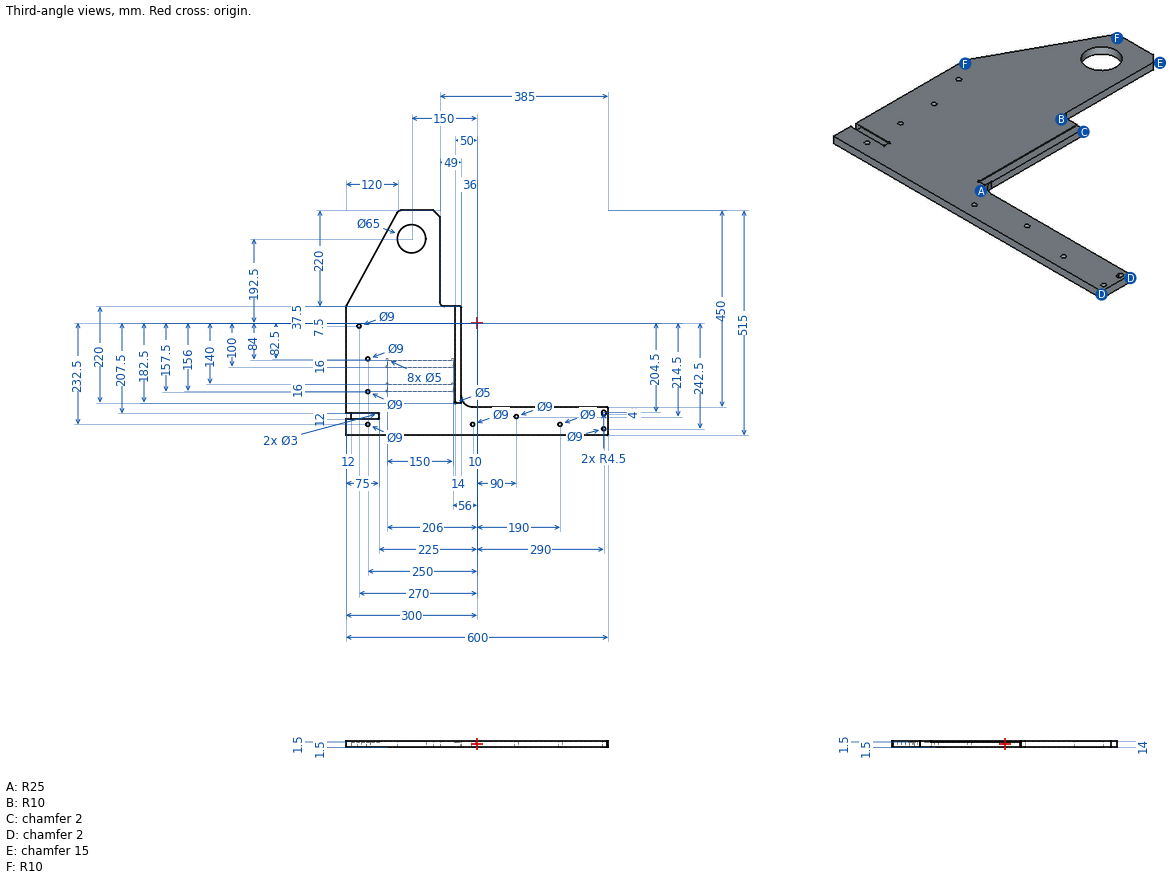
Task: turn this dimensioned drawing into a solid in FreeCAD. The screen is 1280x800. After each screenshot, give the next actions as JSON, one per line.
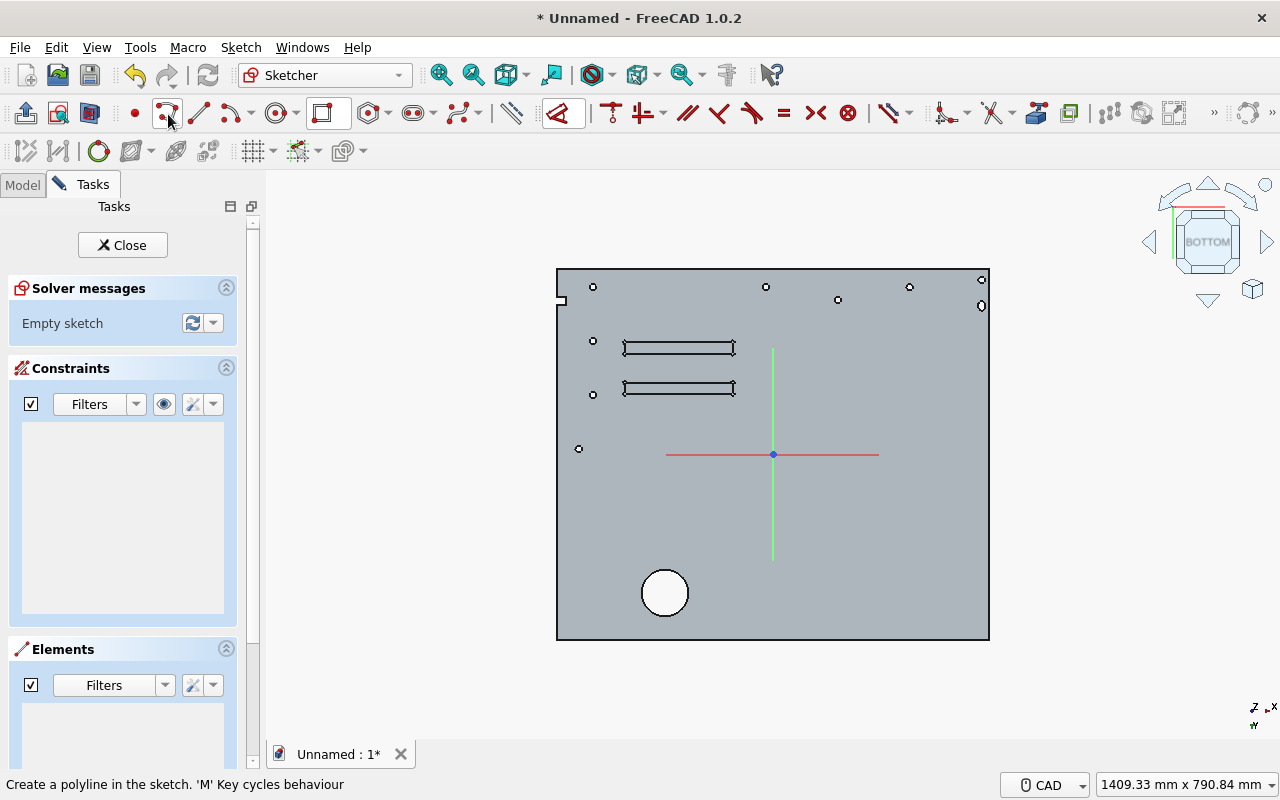
{"action": "left_click", "coordinate": [747, 481]}
{"action": "left_click", "coordinate": [712, 481]}
{"action": "left_click", "coordinate": [712, 640]}
{"action": "left_click", "coordinate": [989, 640]}
{"action": "left_click", "coordinate": [989, 316]}
{"action": "left_click", "coordinate": [747, 316]}
{"action": "left_click", "coordinate": [747, 482]}
{"action": "key", "text": "Escape"}
{"action": "key", "text": "Escape"}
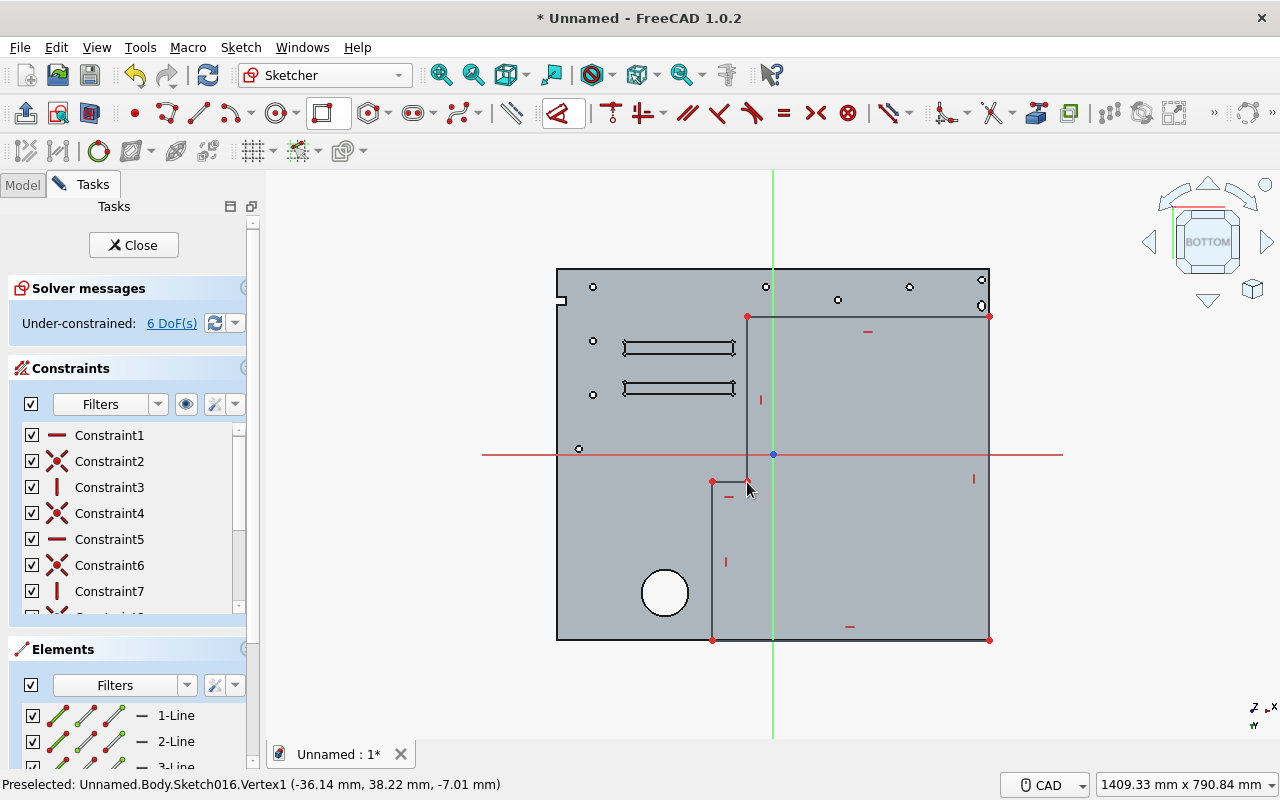
{"action": "scroll", "coordinate": [736, 482], "scroll_direction": "up", "scroll_amount": 2}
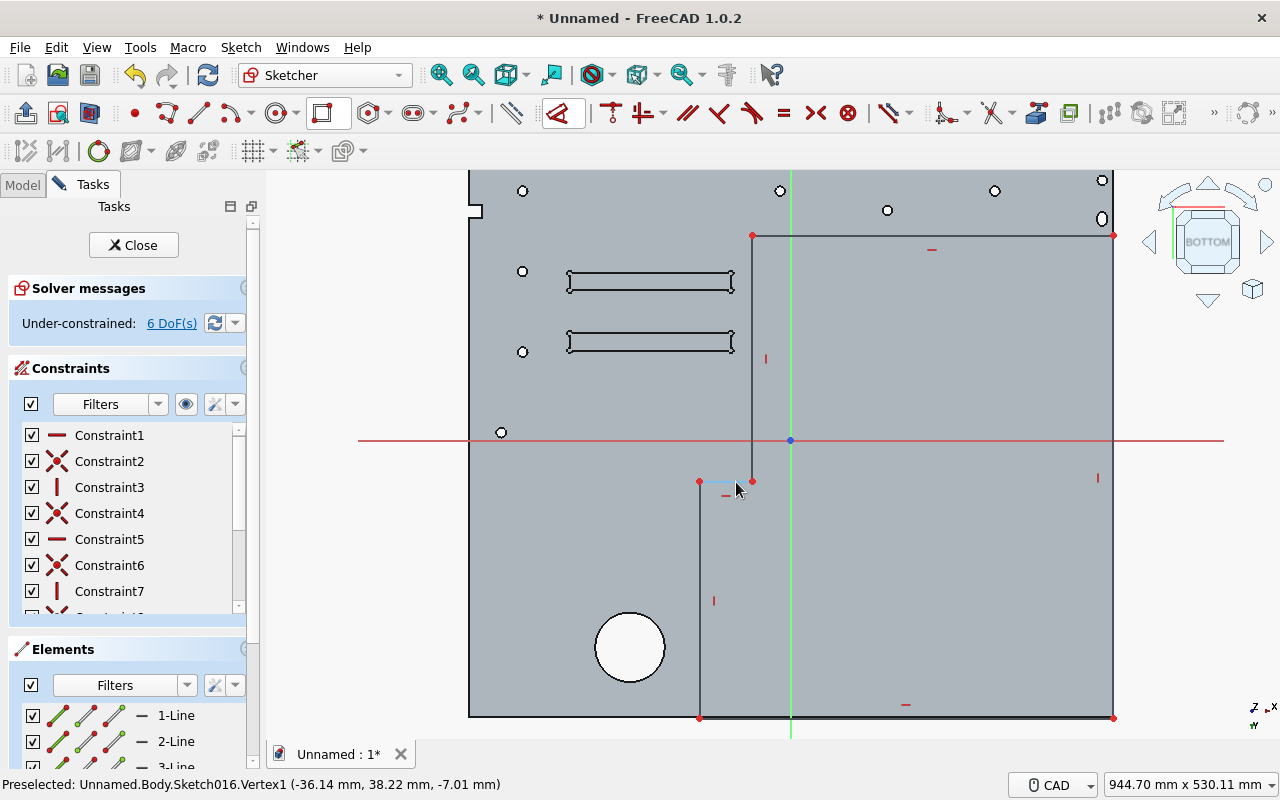
{"action": "left_click", "coordinate": [737, 482]}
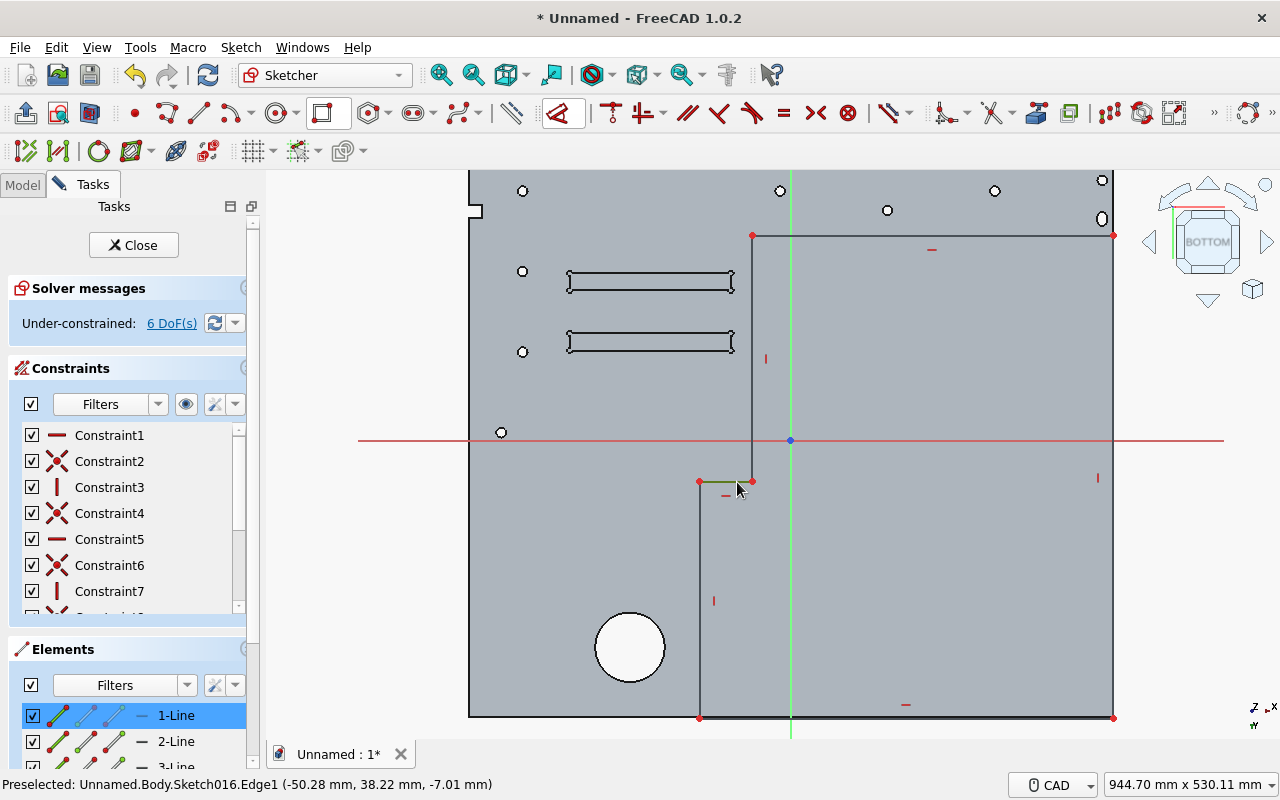
{"action": "left_click", "coordinate": [580, 114]}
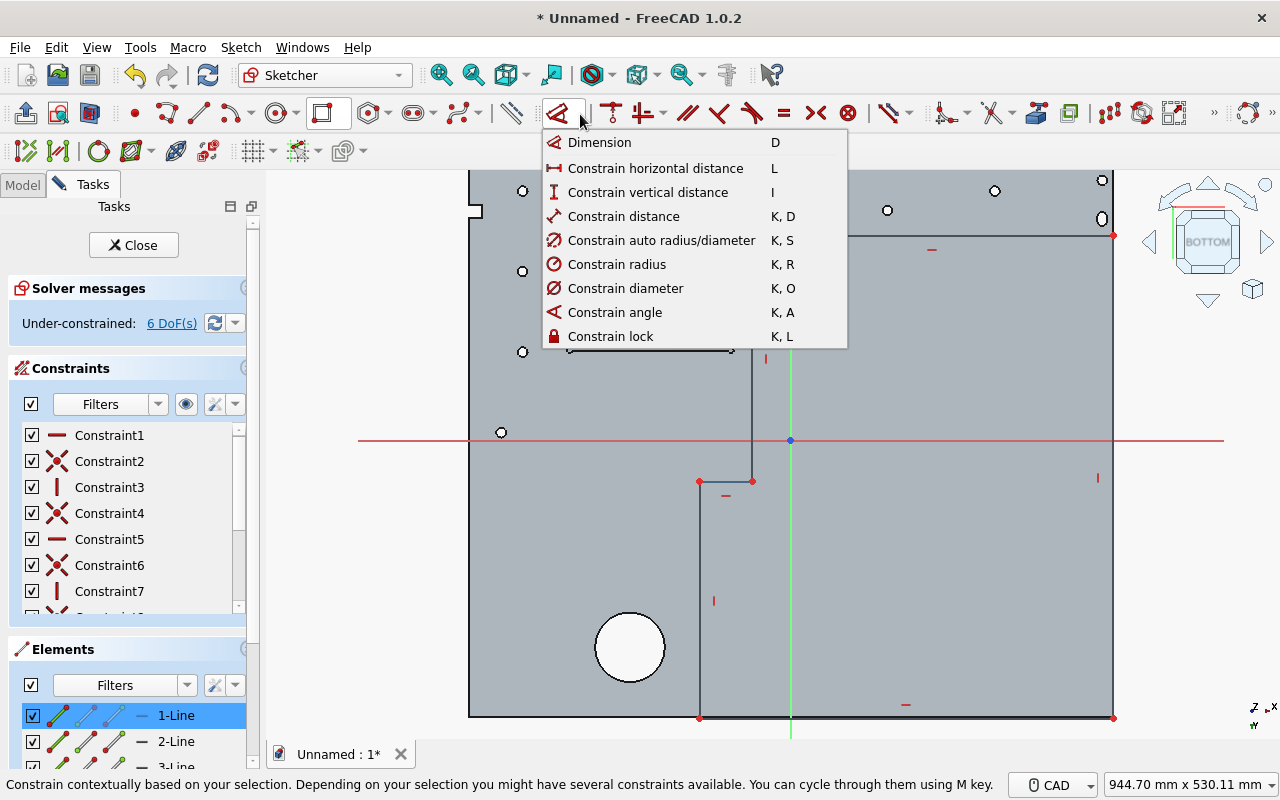
{"action": "left_click", "coordinate": [695, 168]}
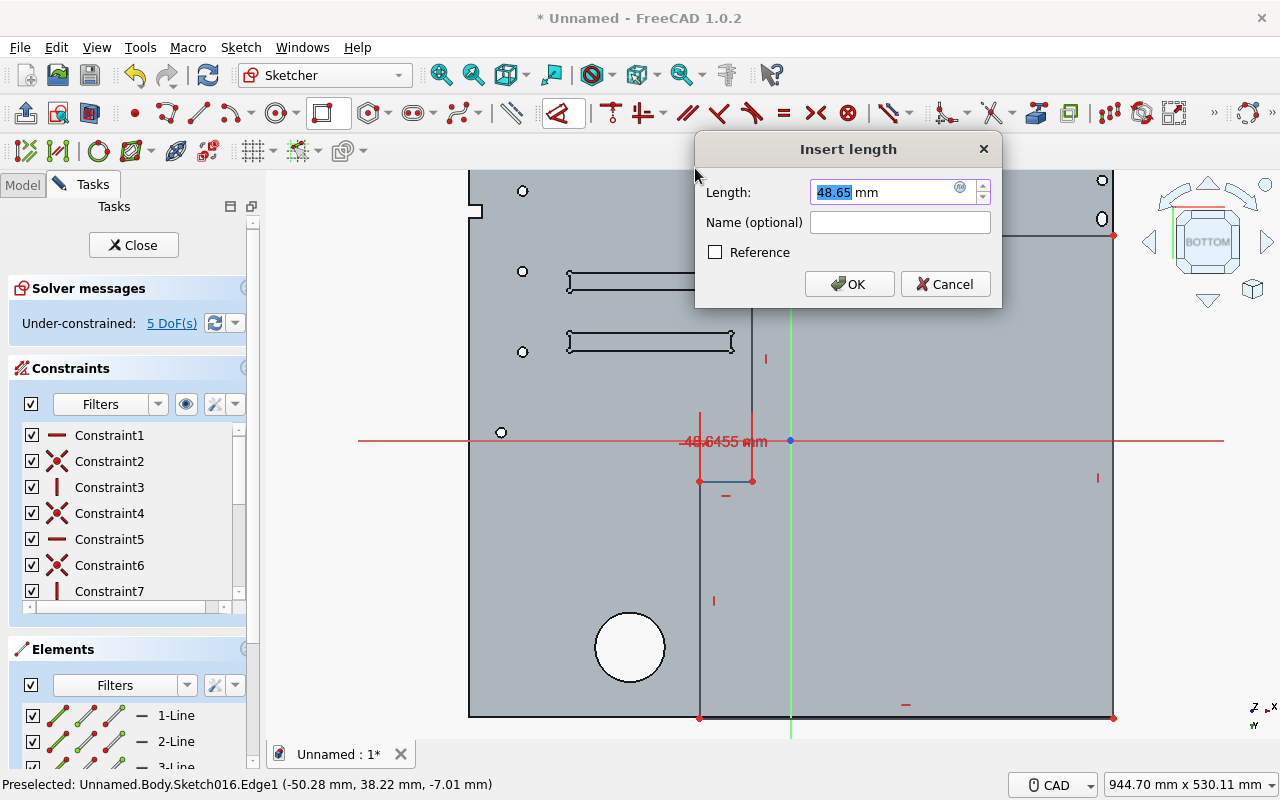
{"action": "type", "text": "49"}
{"action": "key", "text": "Return"}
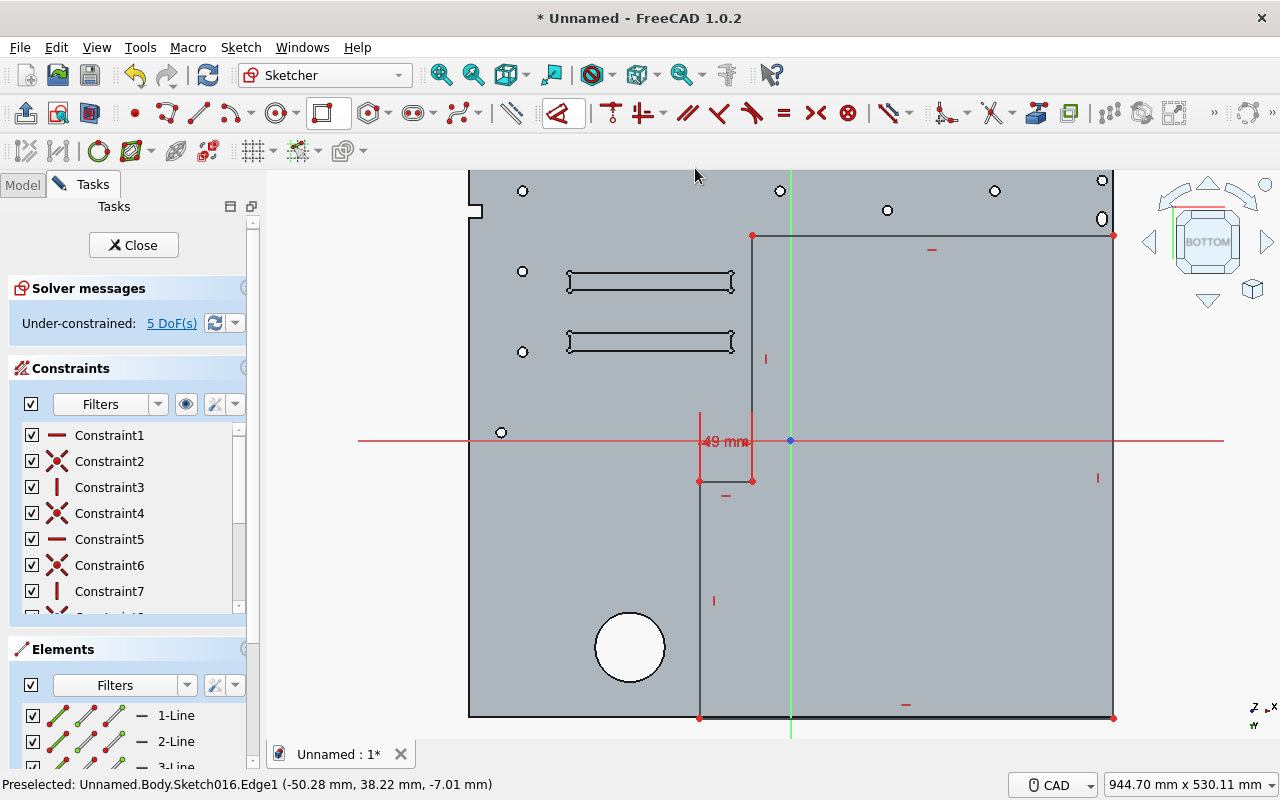
{"action": "left_click", "coordinate": [700, 553]}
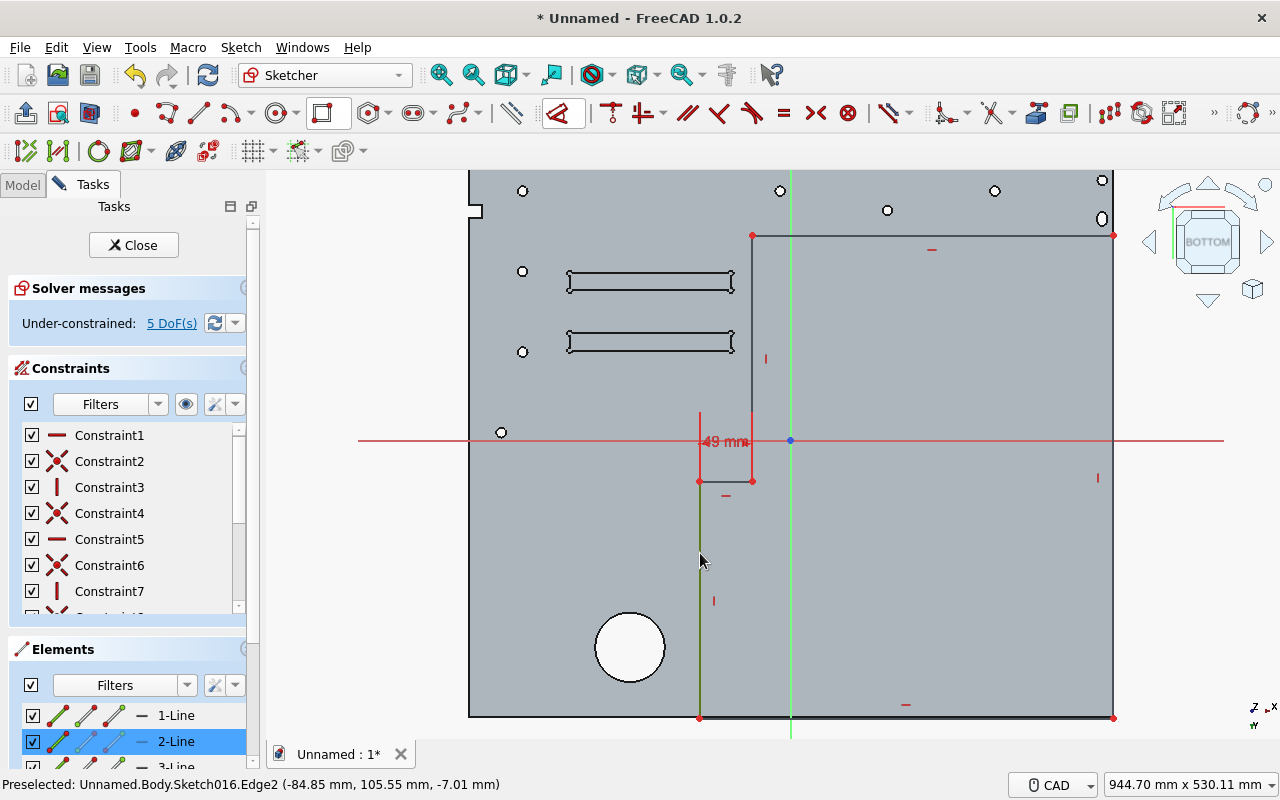
{"action": "left_click", "coordinate": [580, 114]}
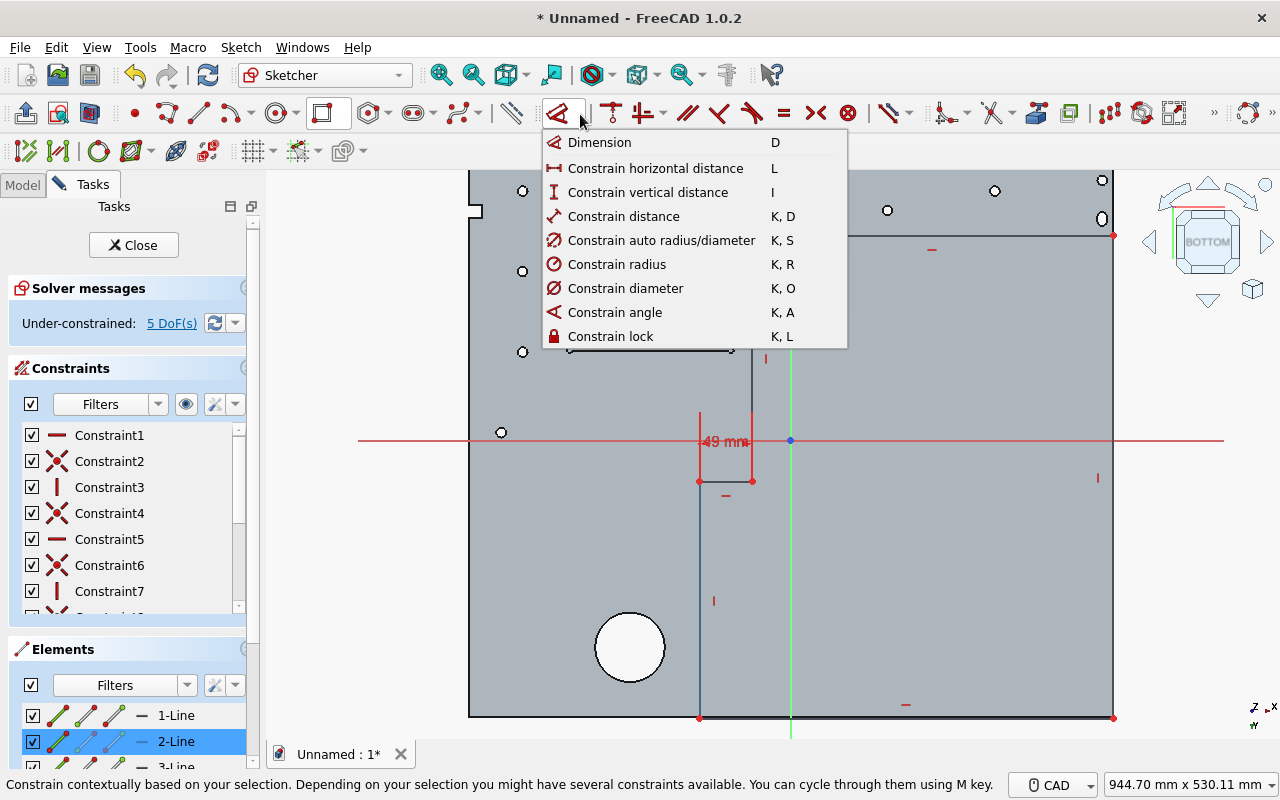
{"action": "left_click", "coordinate": [695, 192]}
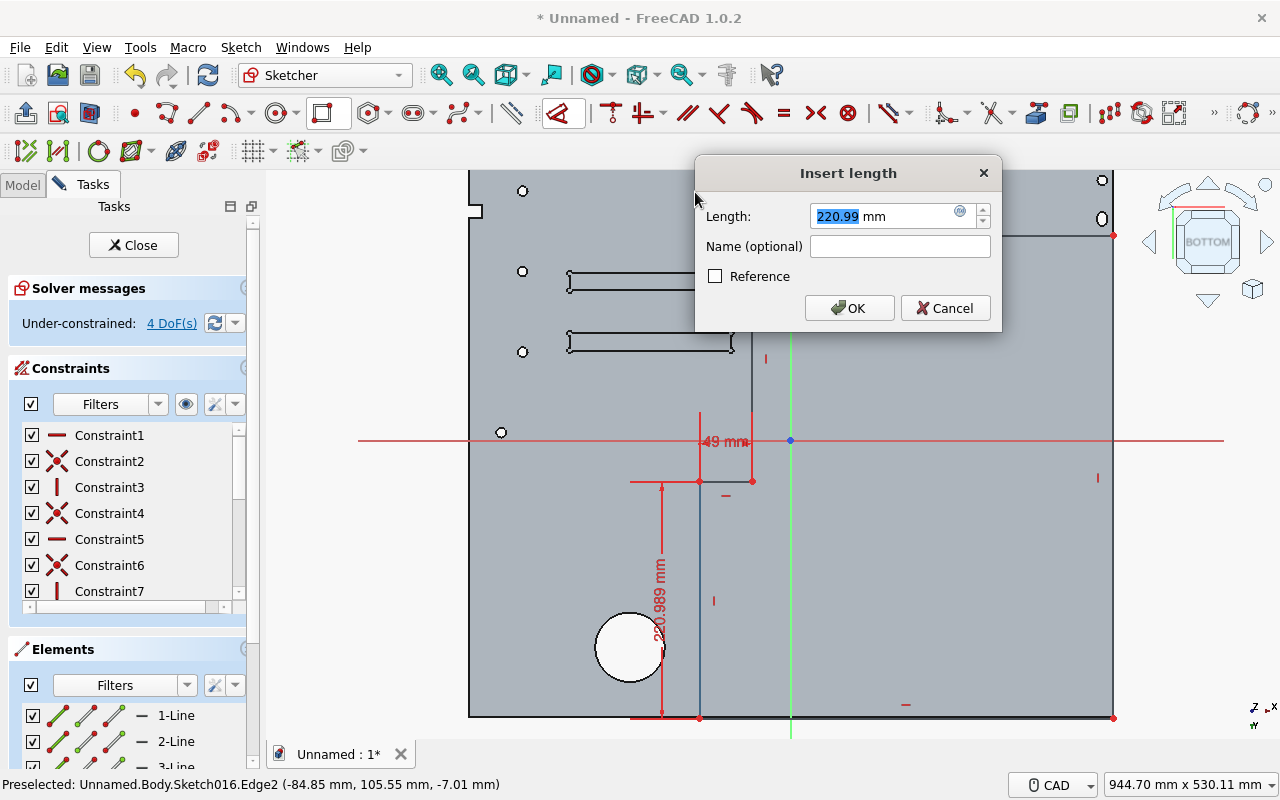
{"action": "type", "text": "220"}
{"action": "key", "text": "Return"}